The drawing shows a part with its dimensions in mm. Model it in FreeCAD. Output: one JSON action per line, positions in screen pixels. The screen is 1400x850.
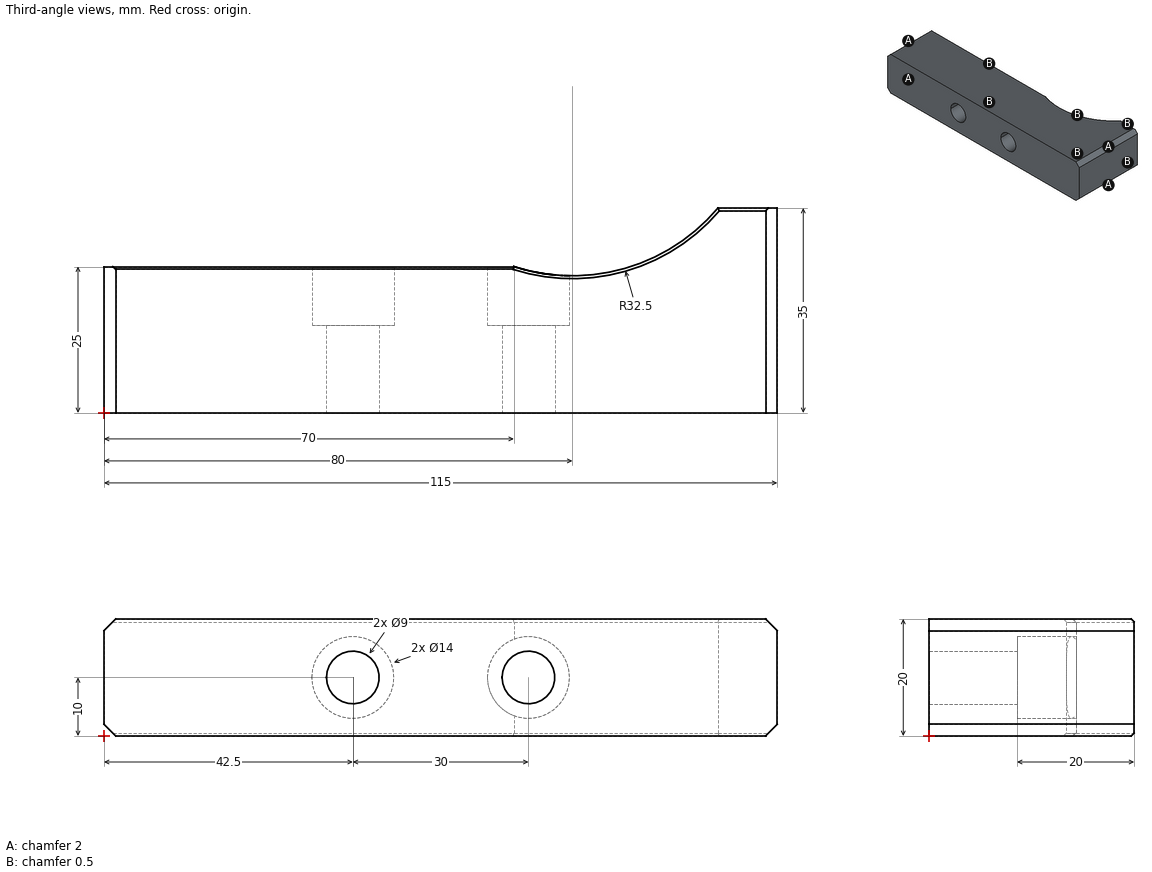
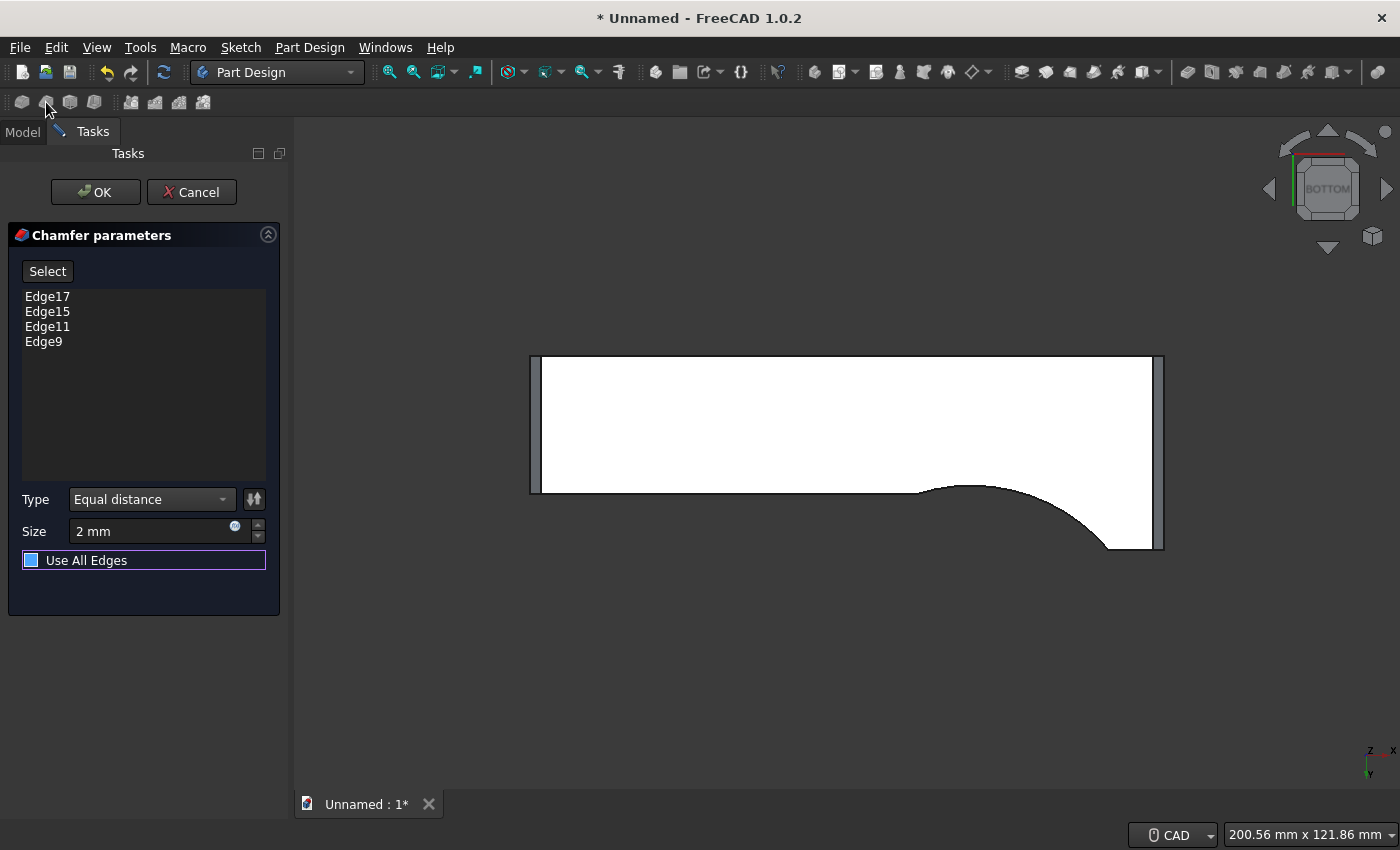
{"action": "left_click", "coordinate": [96, 192]}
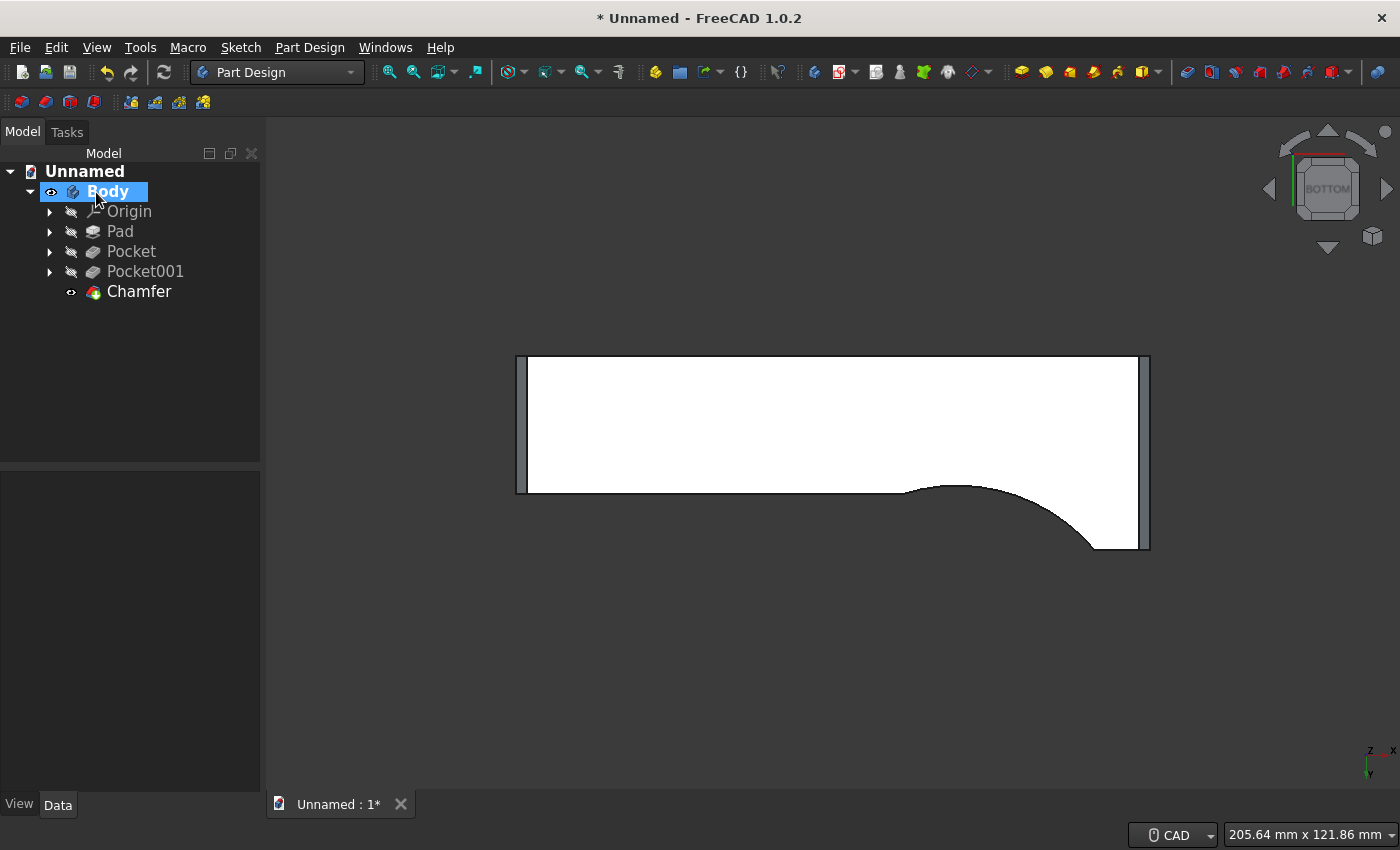
{"action": "left_click", "coordinate": [714, 493]}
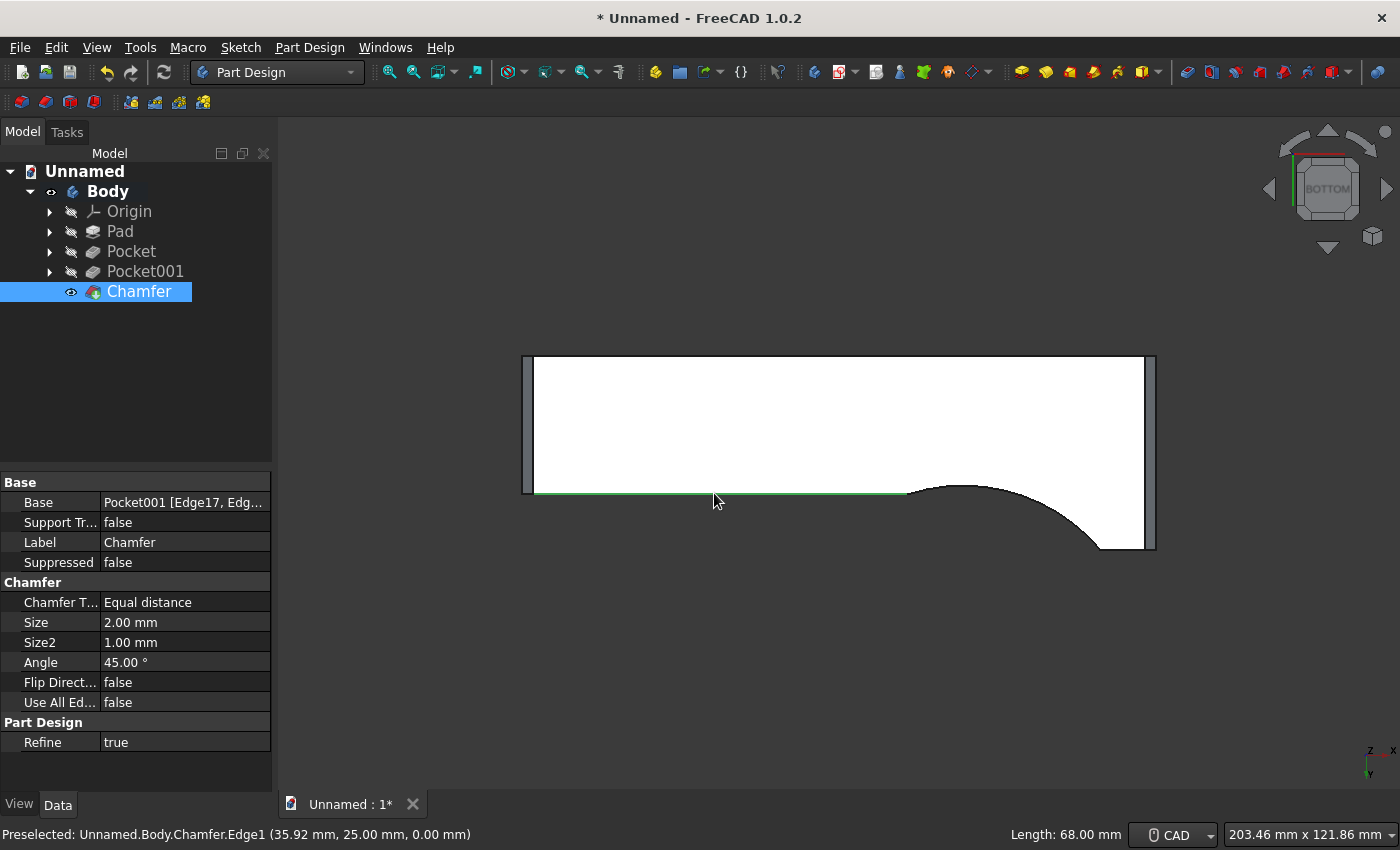
{"action": "left_click", "coordinate": [914, 492], "text": "ctrl"}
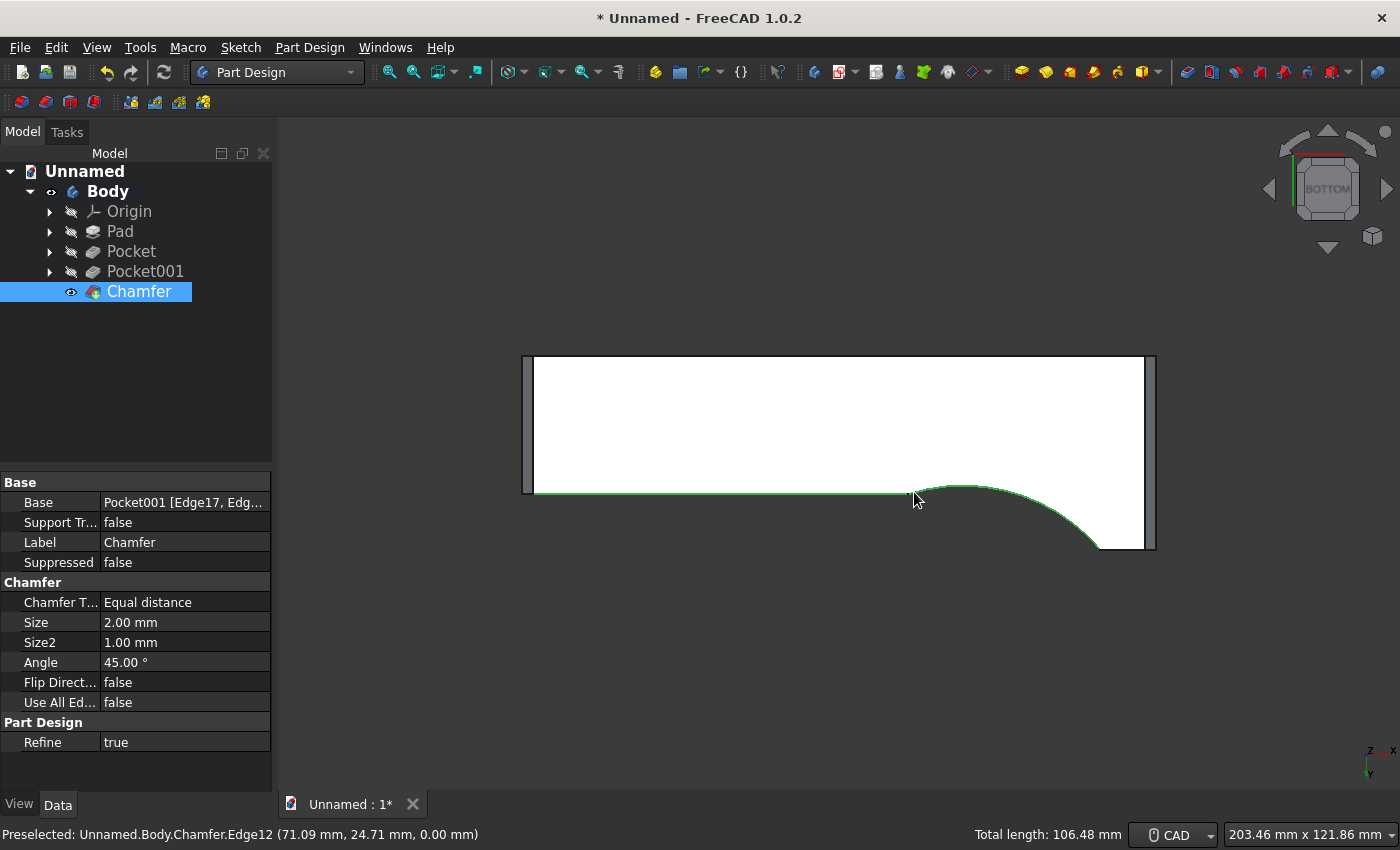
{"action": "key", "text": "0"}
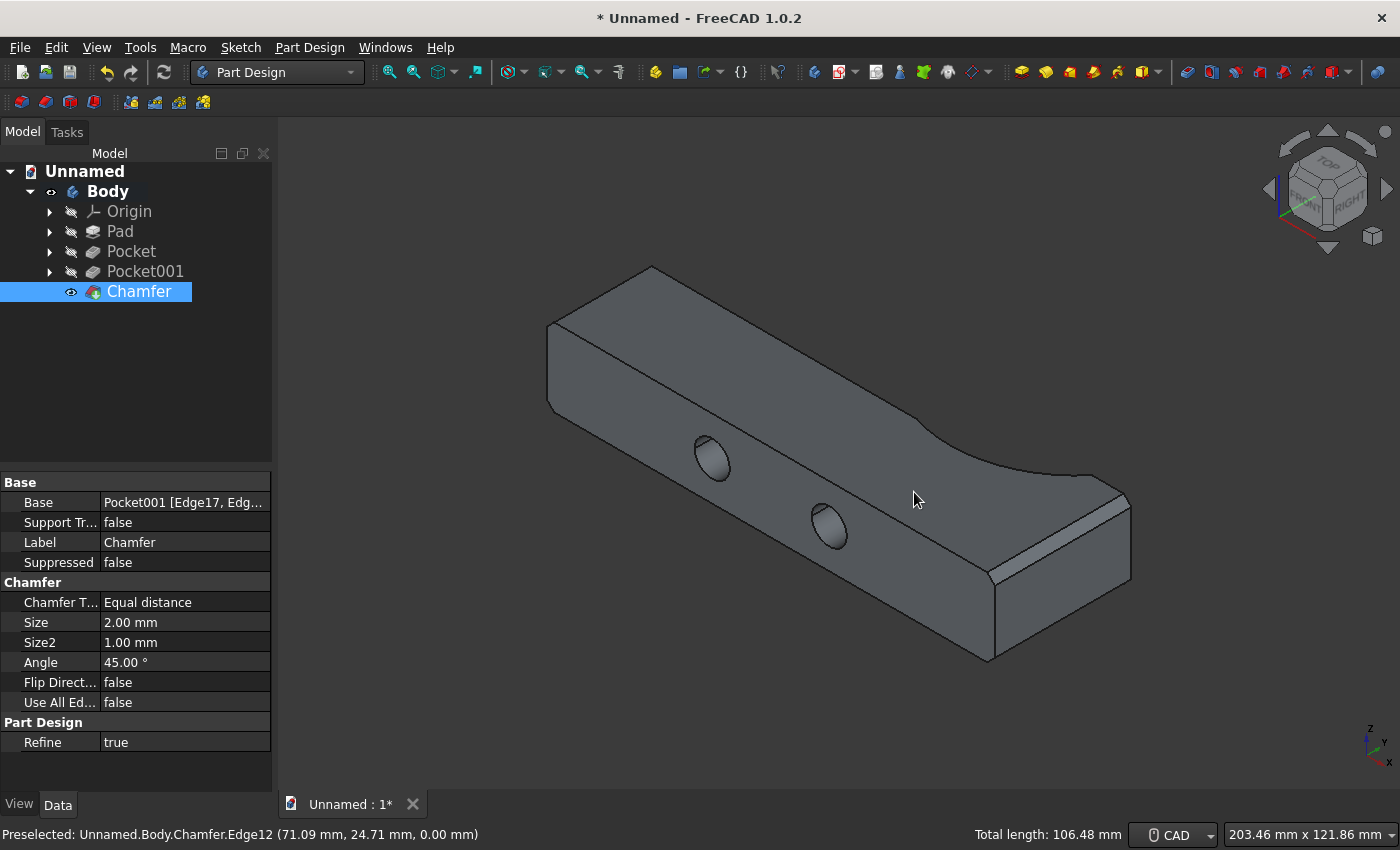
{"action": "key", "text": "2"}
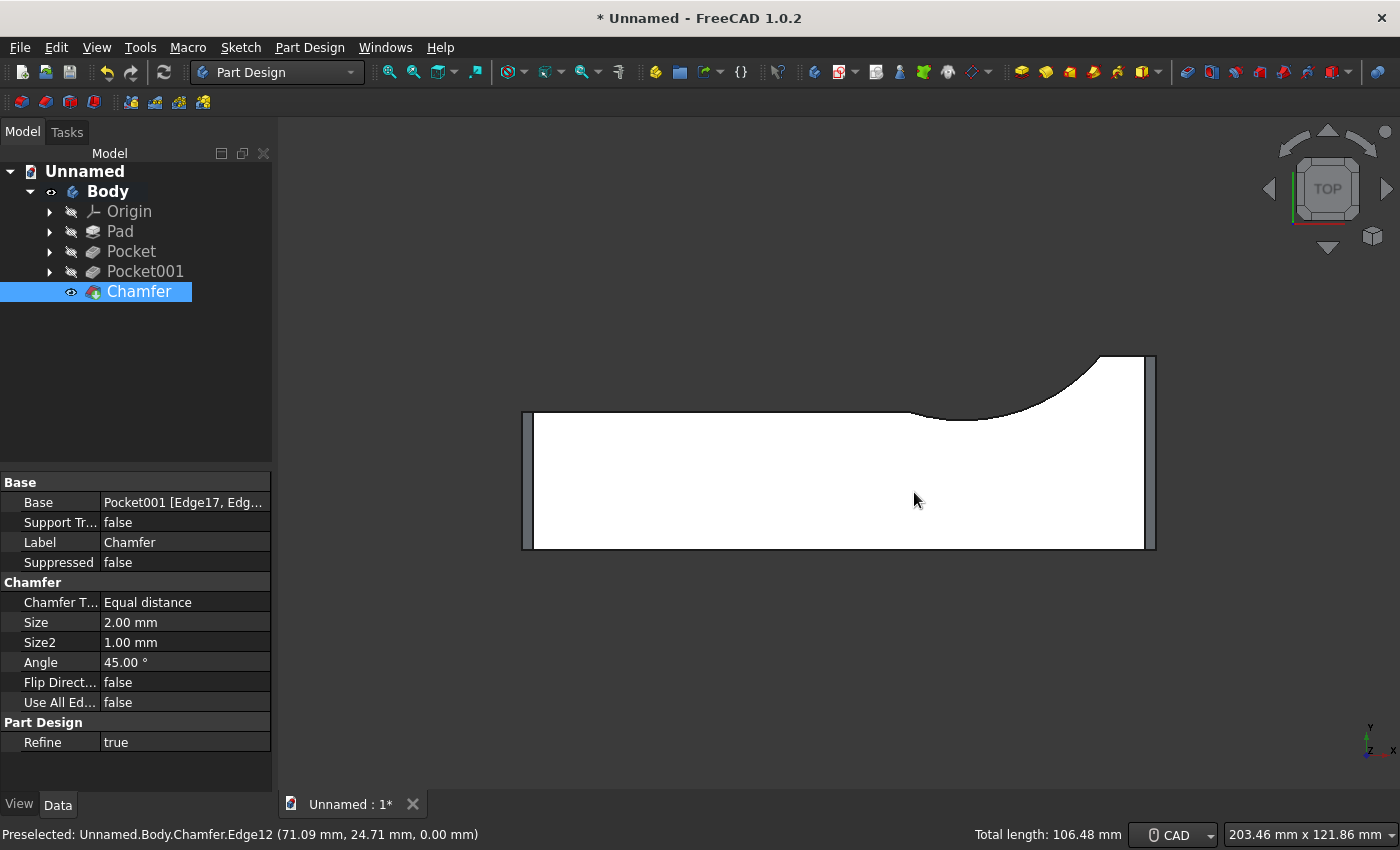
{"action": "left_click", "coordinate": [1012, 412], "text": "ctrl"}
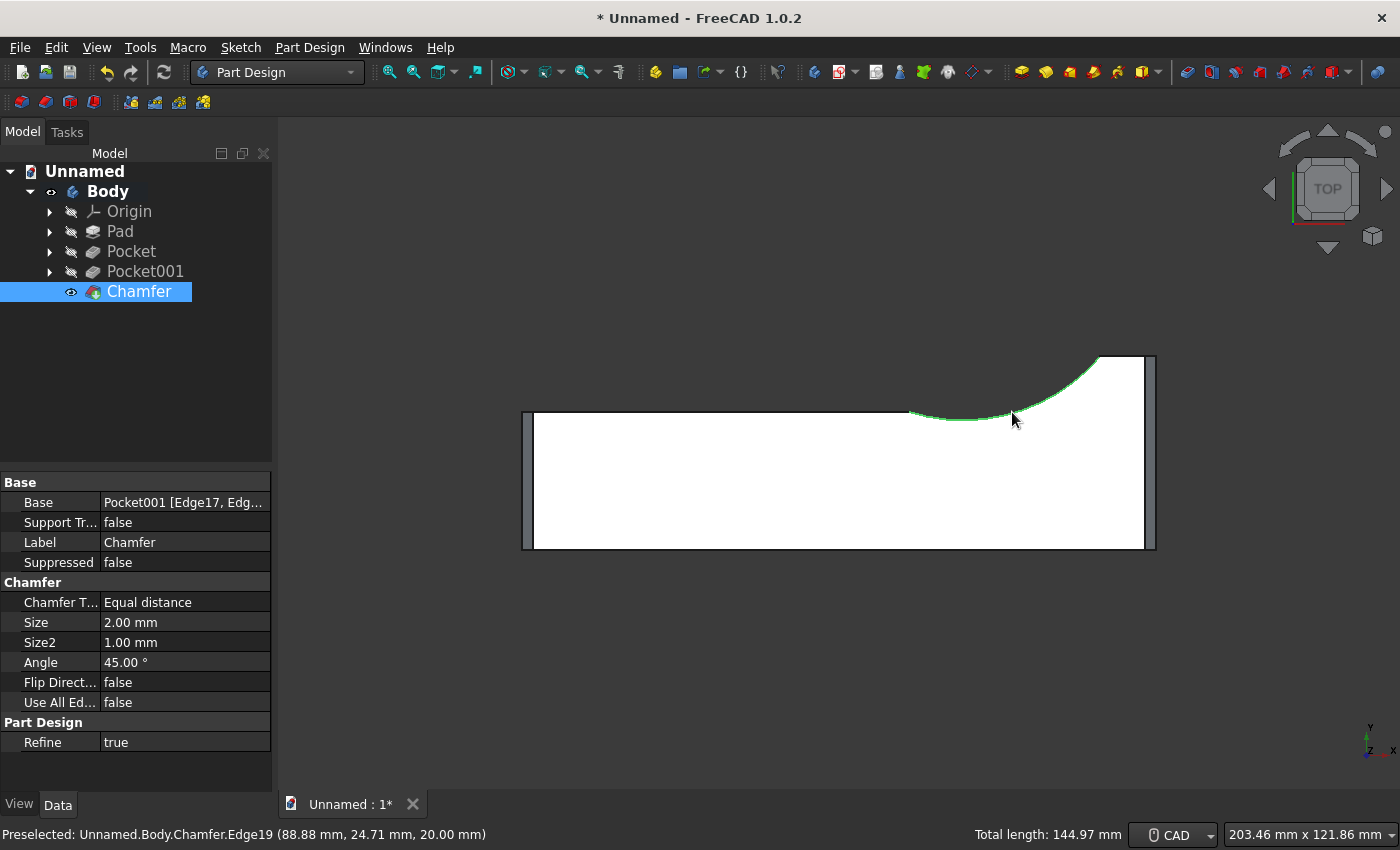
{"action": "left_click", "coordinate": [720, 411], "text": "ctrl"}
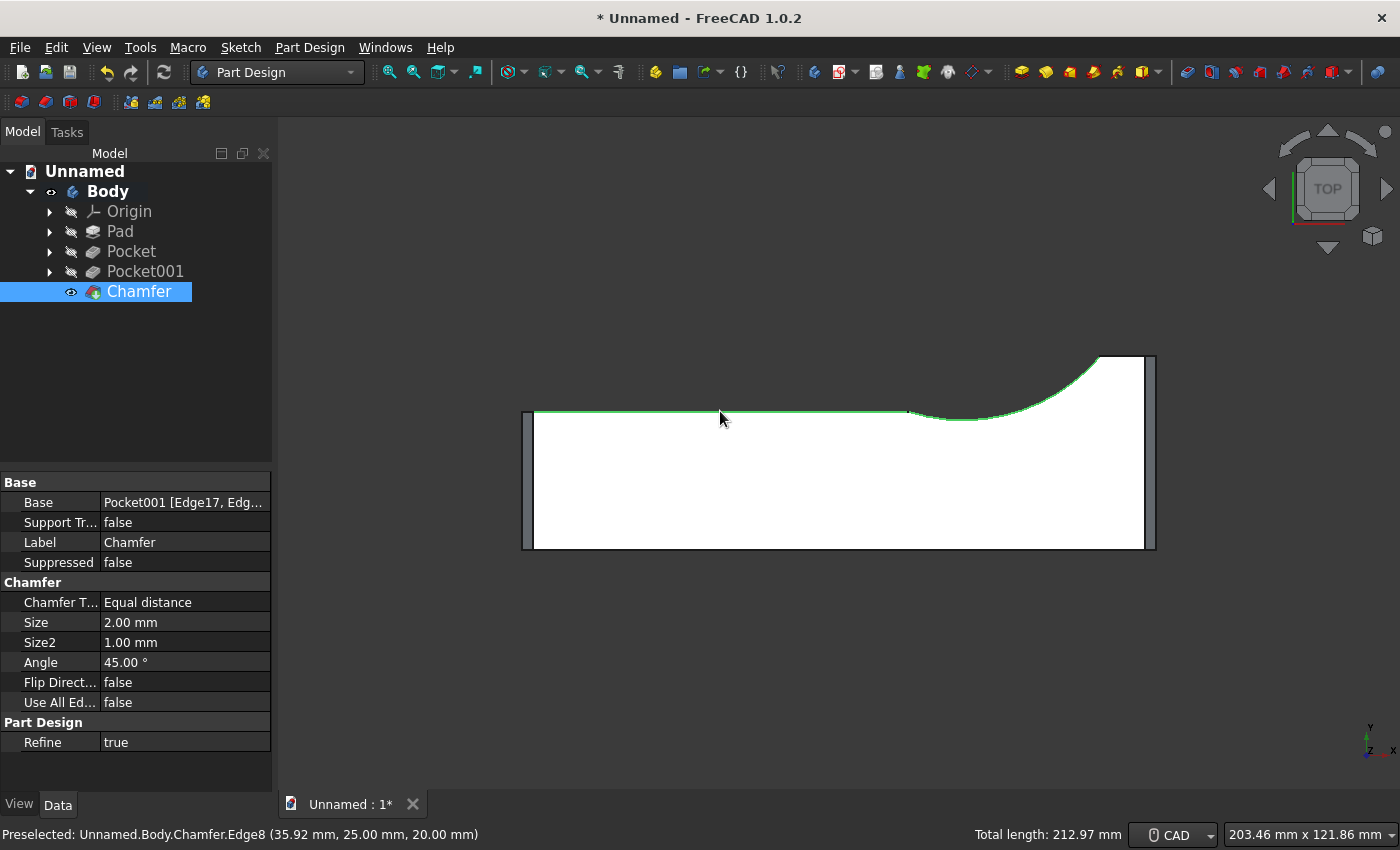
{"action": "left_click", "coordinate": [1123, 355], "text": "ctrl"}